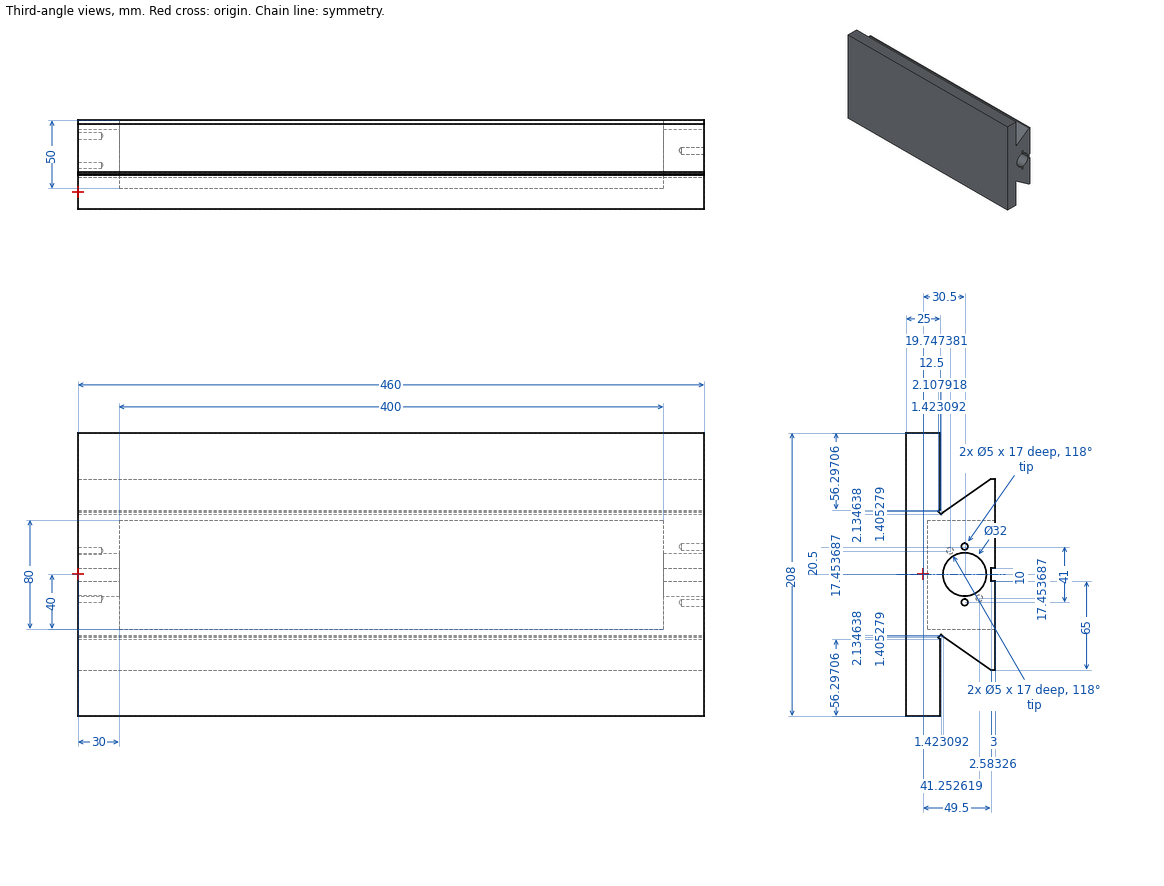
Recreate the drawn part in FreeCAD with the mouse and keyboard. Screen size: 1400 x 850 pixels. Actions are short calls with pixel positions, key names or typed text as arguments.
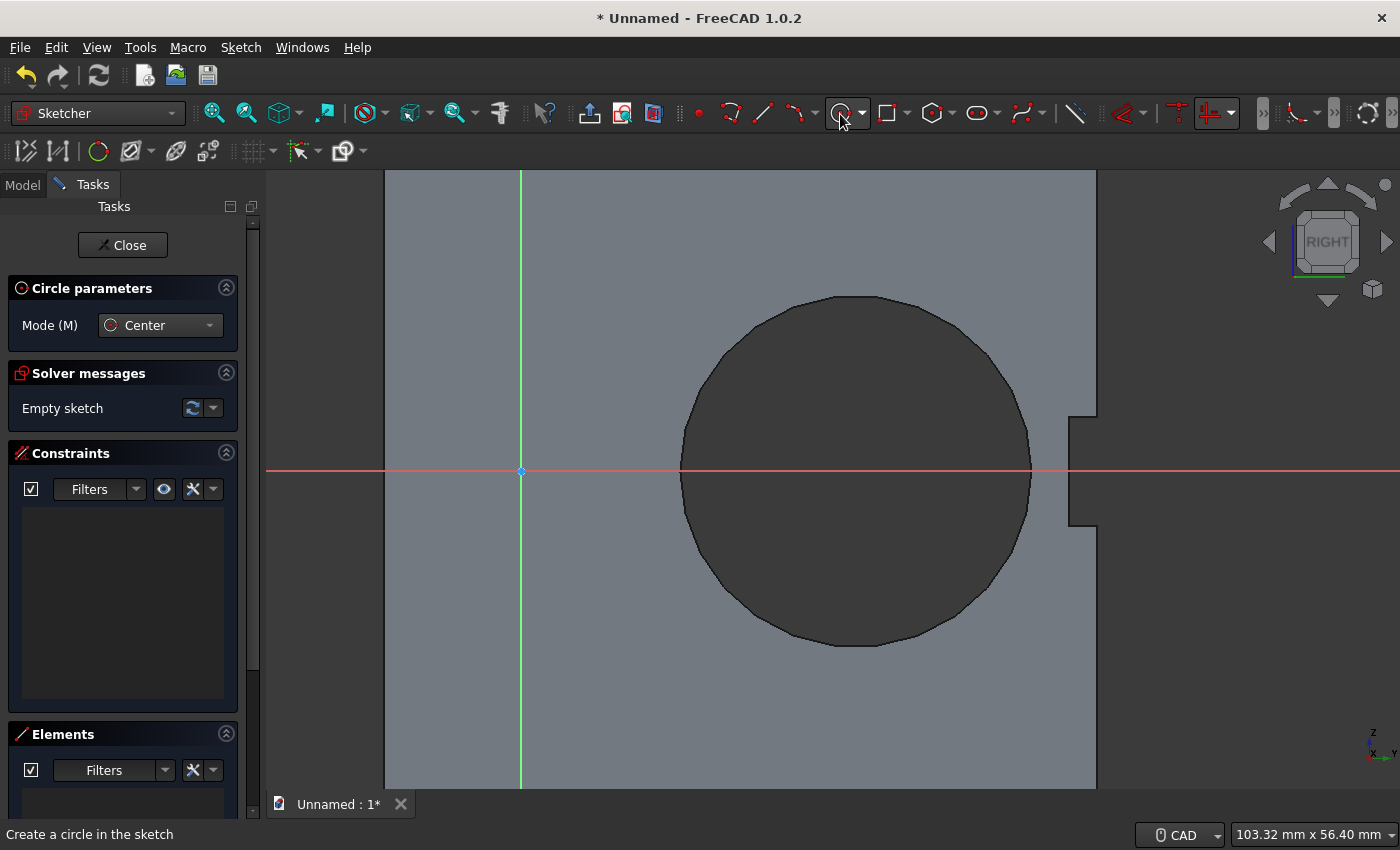
click(738, 280)
move(757, 261)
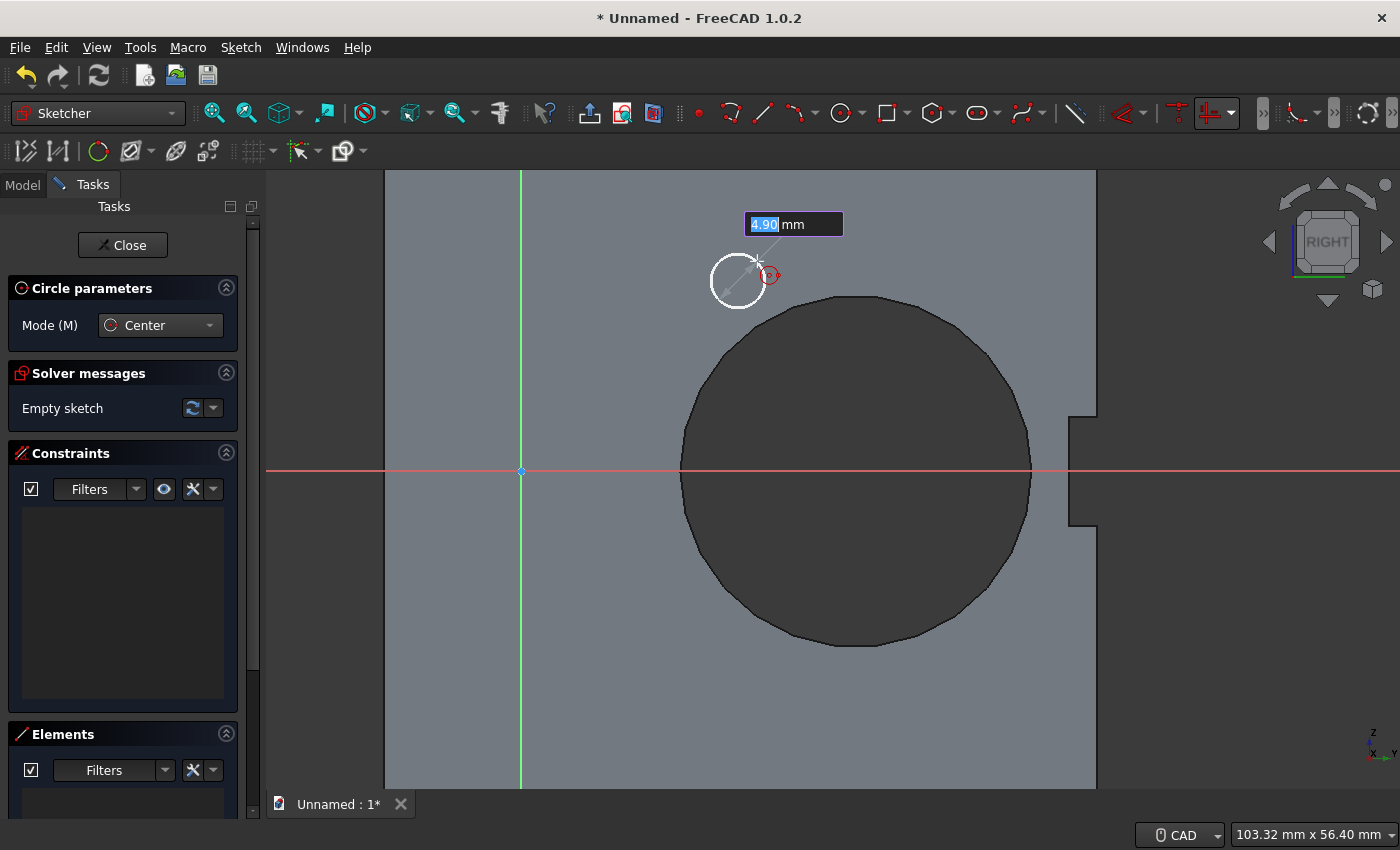
text(5)
key(Return)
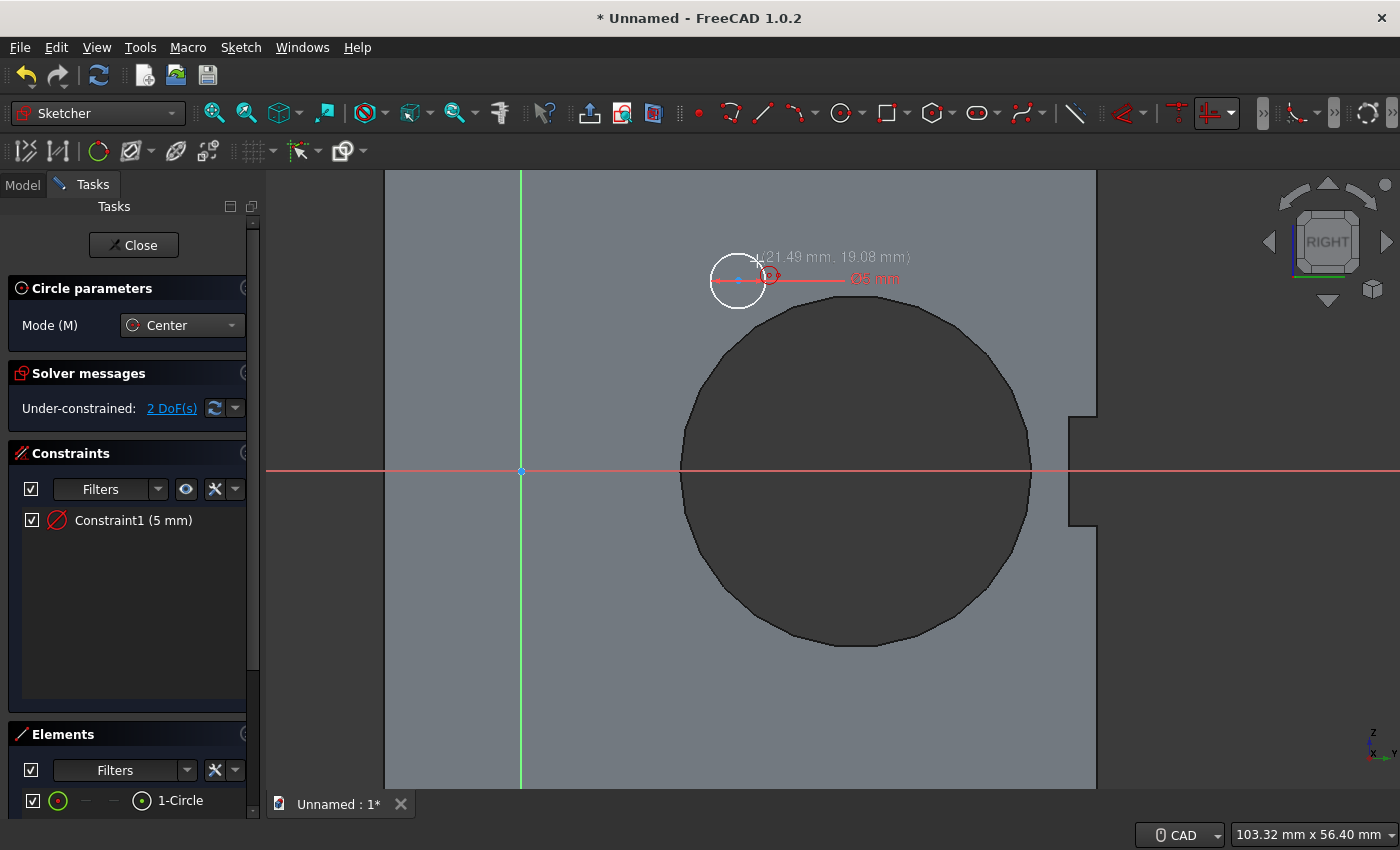
click(974, 663)
move(993, 644)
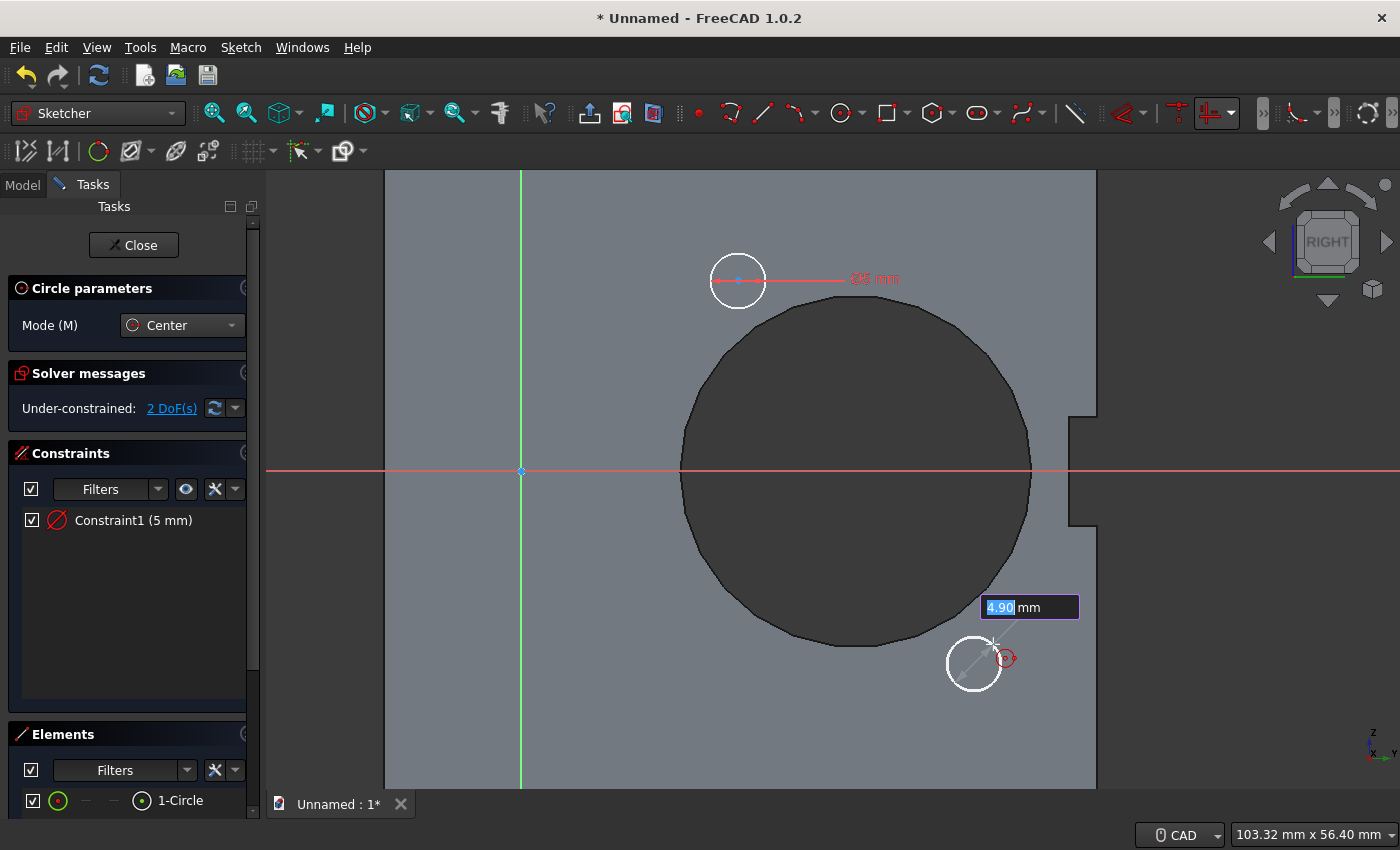
text(5)
key(Return)
key(Escape)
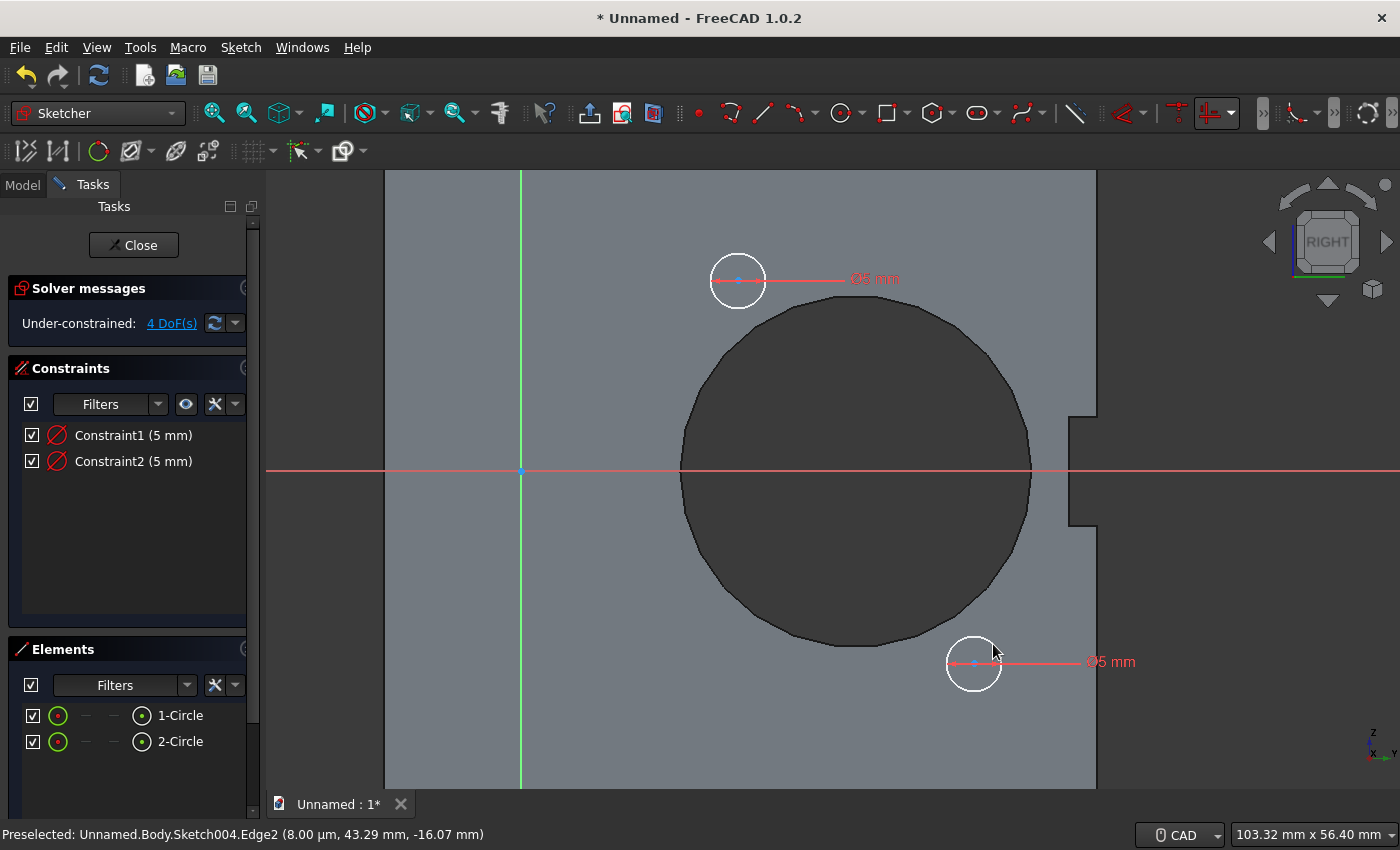
click(1122, 114)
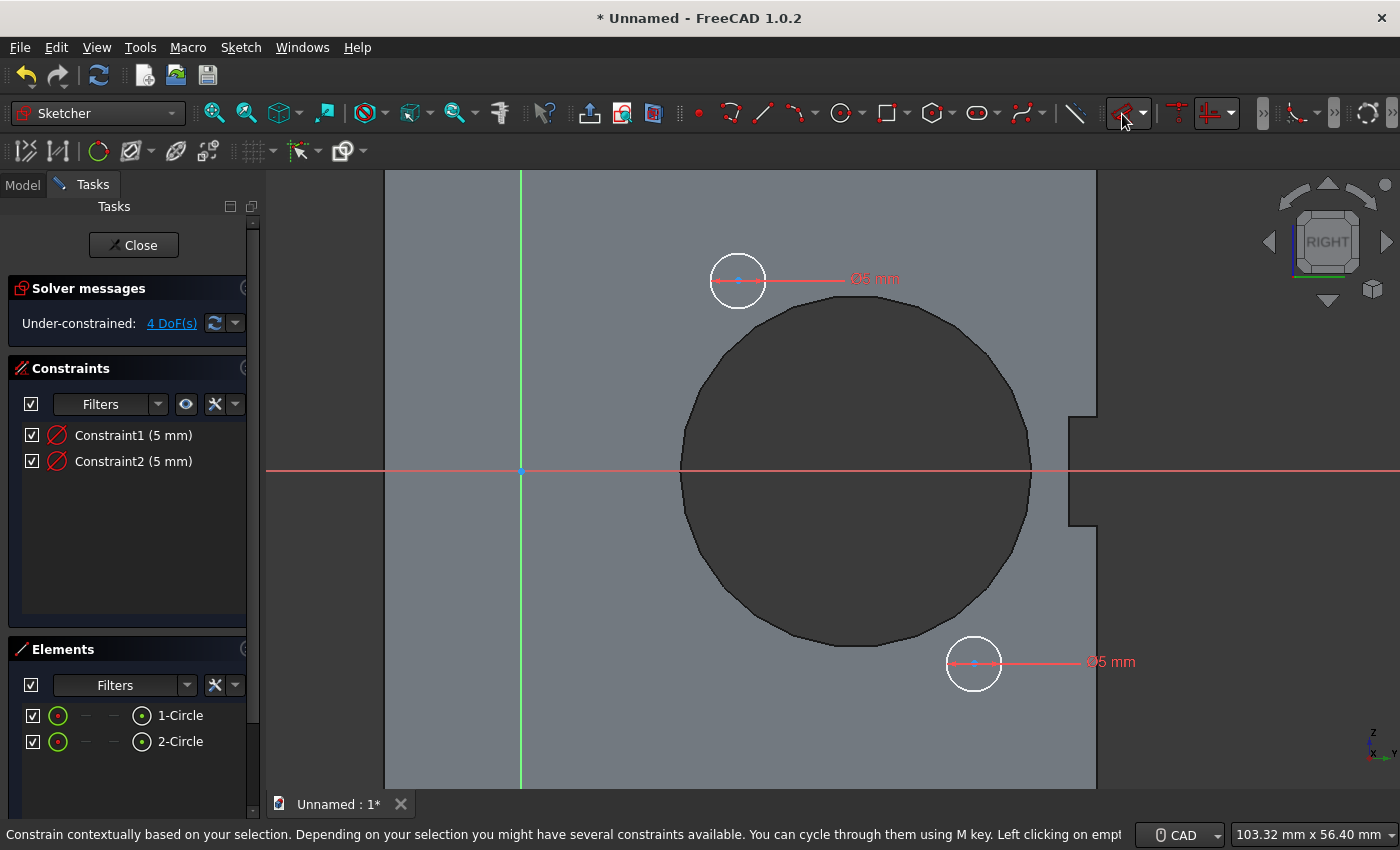
click(738, 281)
click(630, 247)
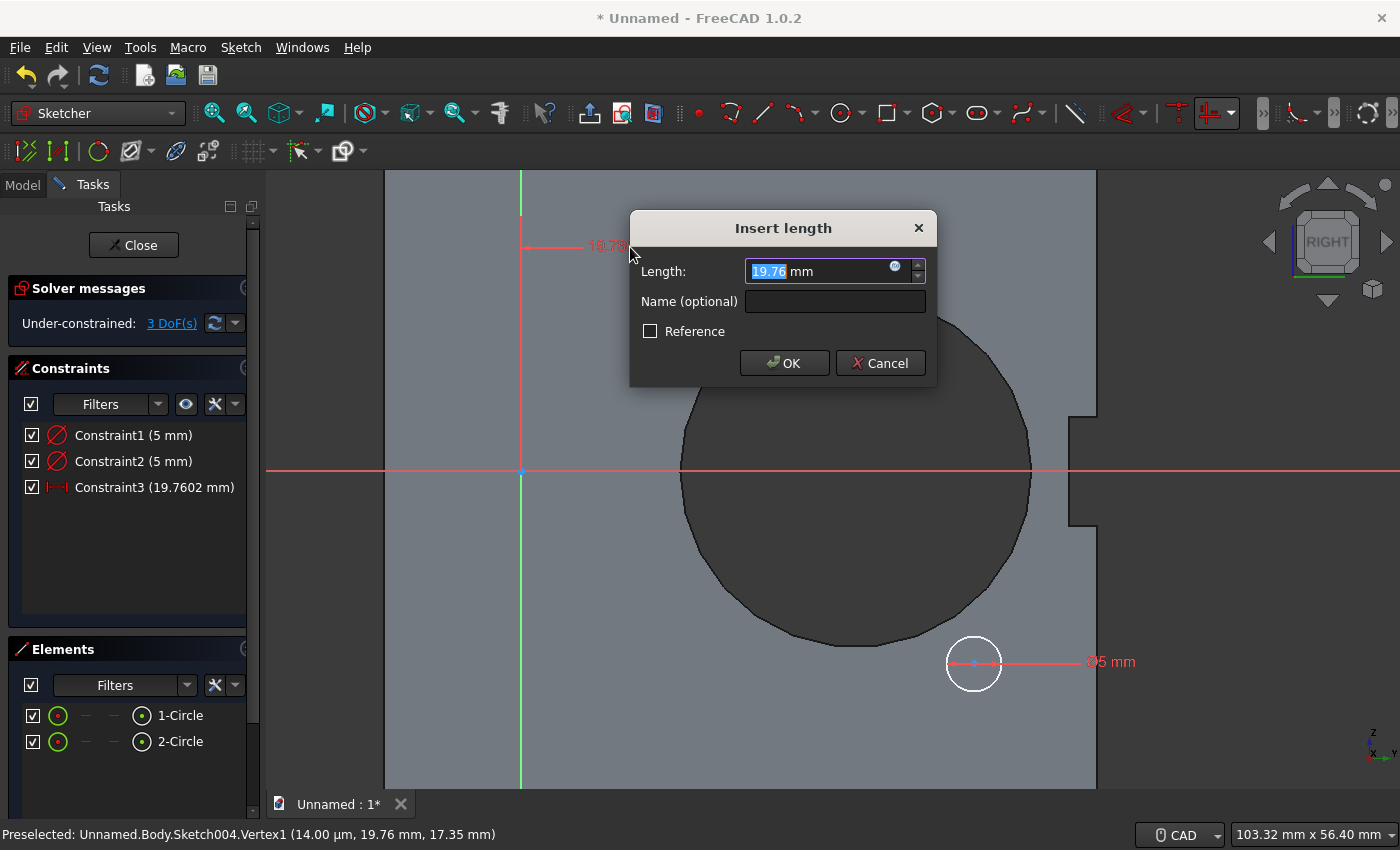
text(19.747381)
key(Return)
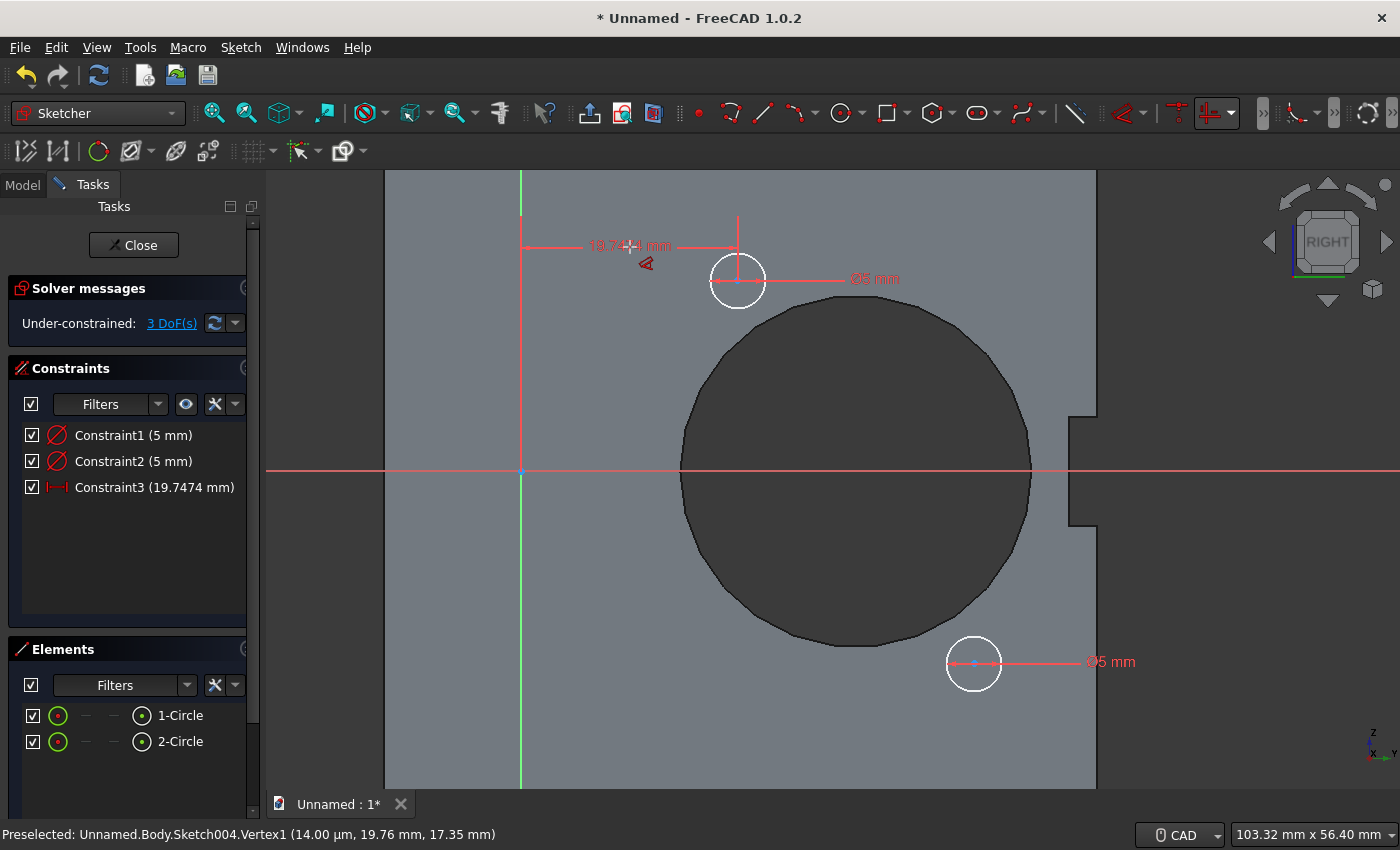
click(738, 281)
click(487, 376)